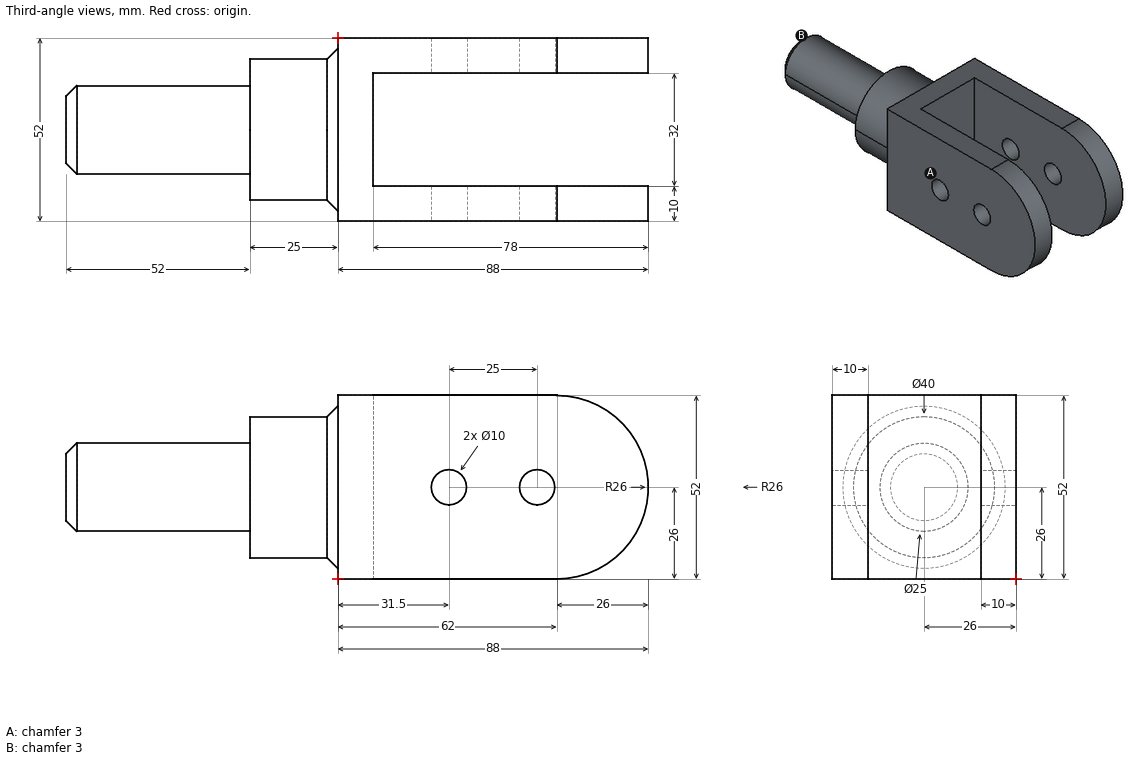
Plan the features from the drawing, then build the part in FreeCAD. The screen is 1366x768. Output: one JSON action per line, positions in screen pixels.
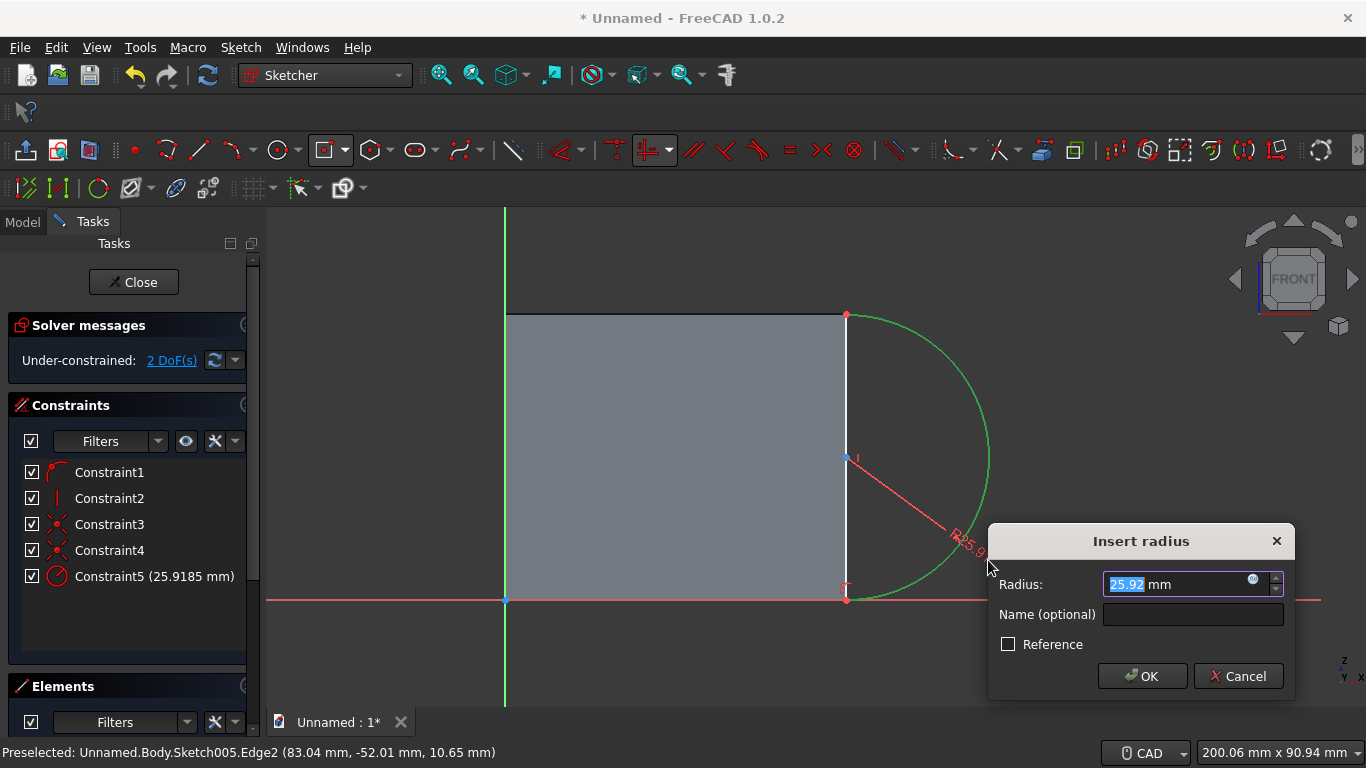
{"action": "type", "text": "26"}
{"action": "key", "text": "Return"}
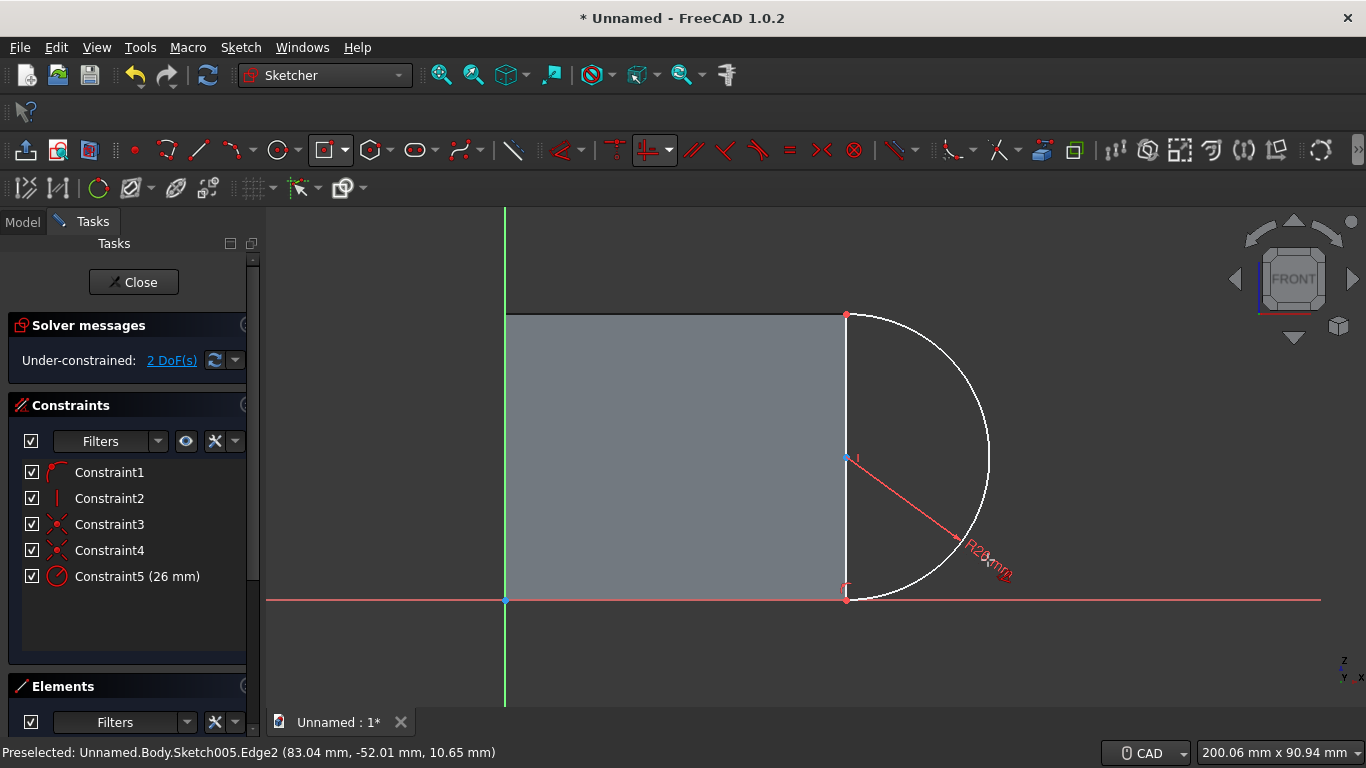
{"action": "left_click", "coordinate": [846, 314]}
{"action": "left_click", "coordinate": [676, 634]}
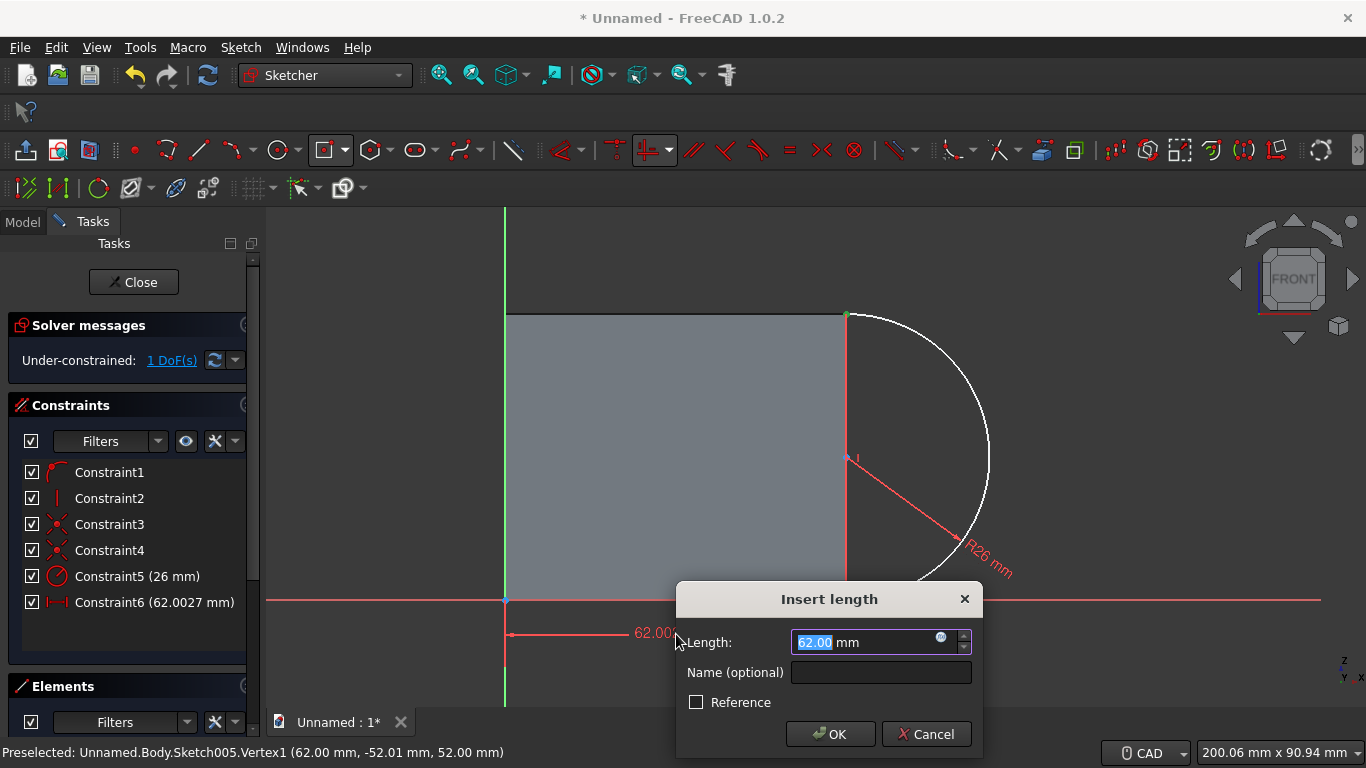
{"action": "type", "text": "62"}
{"action": "key", "text": "Return"}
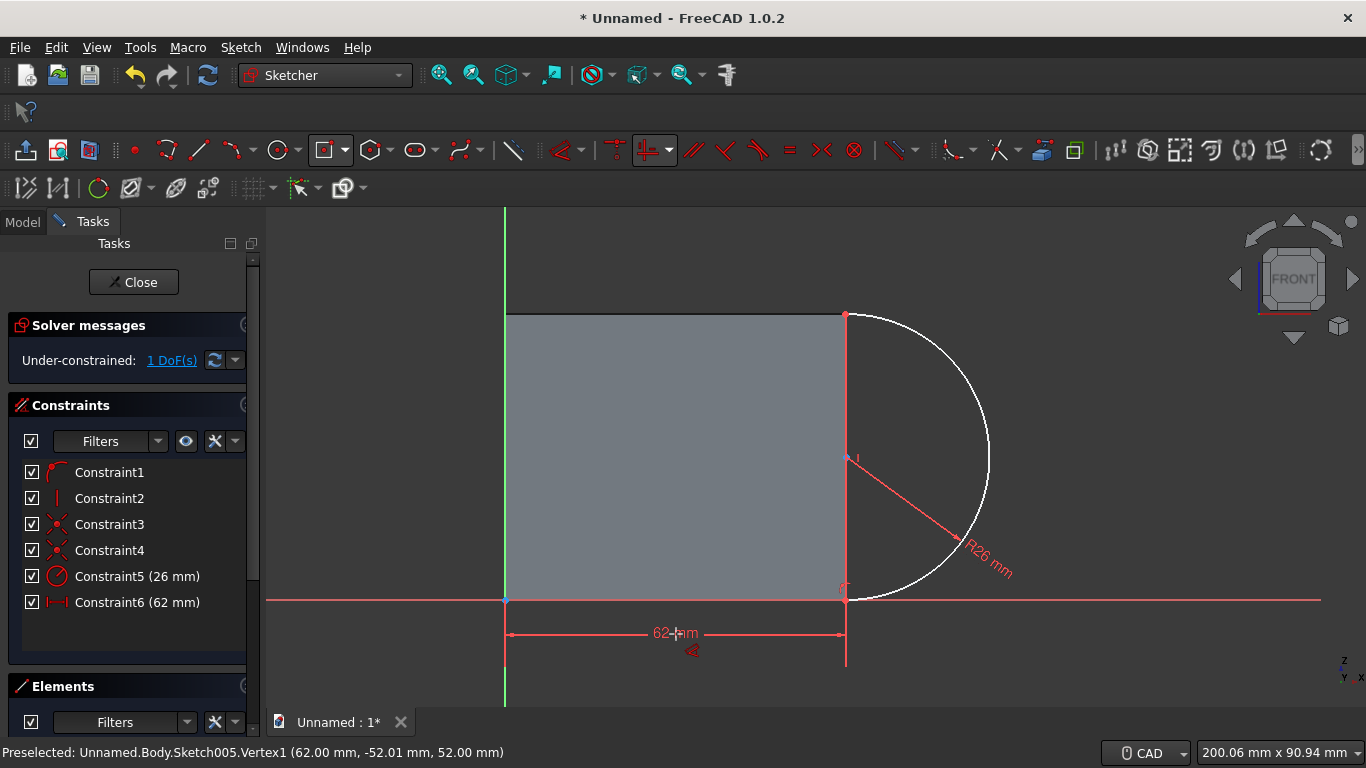
{"action": "left_click", "coordinate": [846, 457]}
{"action": "left_click", "coordinate": [597, 634]}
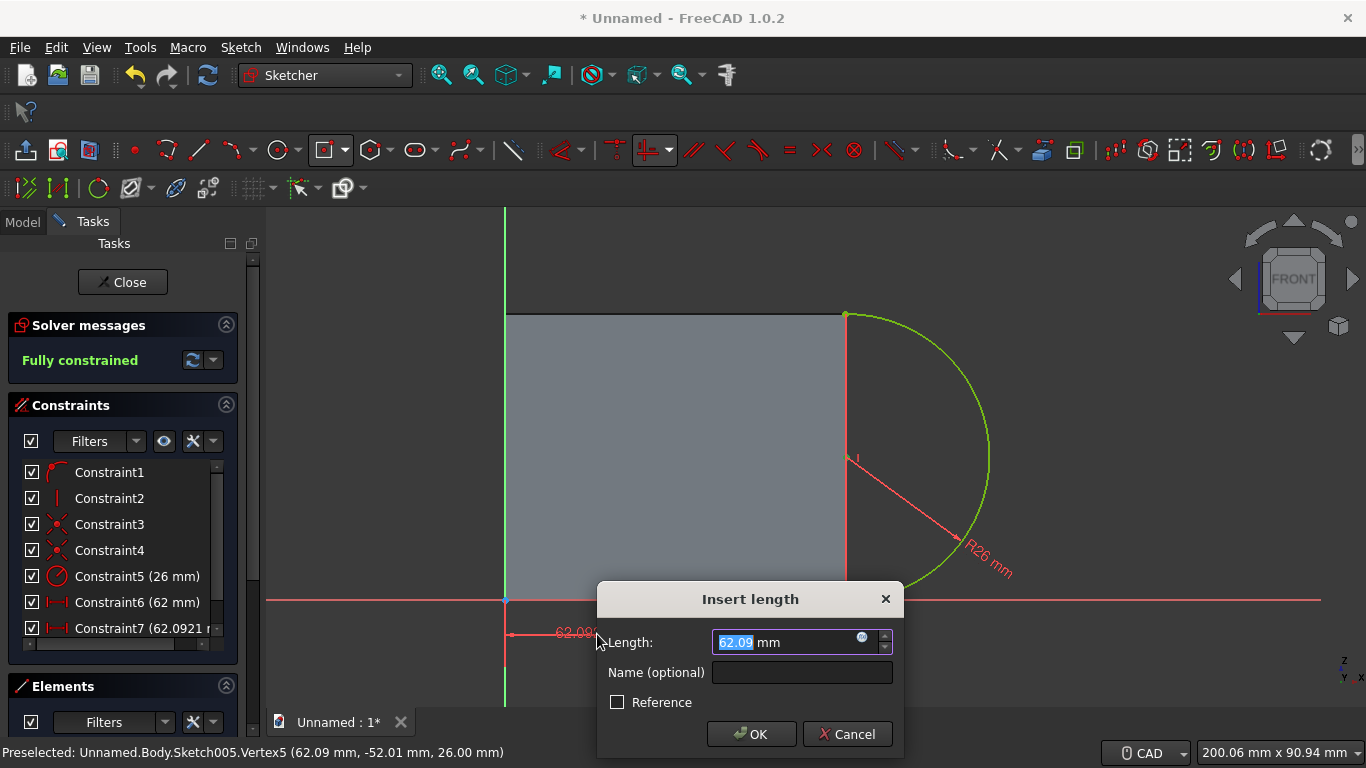
{"action": "type", "text": "62"}
{"action": "key", "text": "Return"}
{"action": "key", "text": "Escape"}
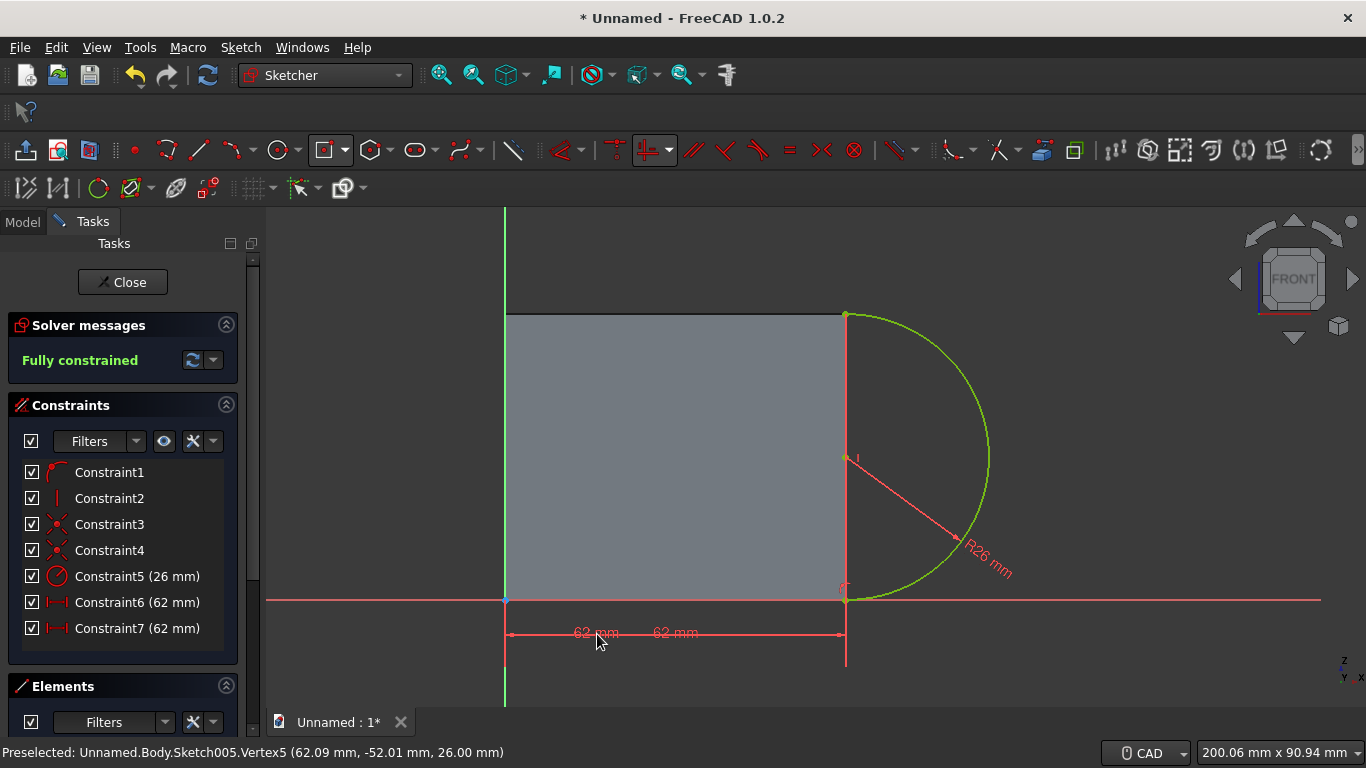
{"action": "left_click", "coordinate": [123, 282]}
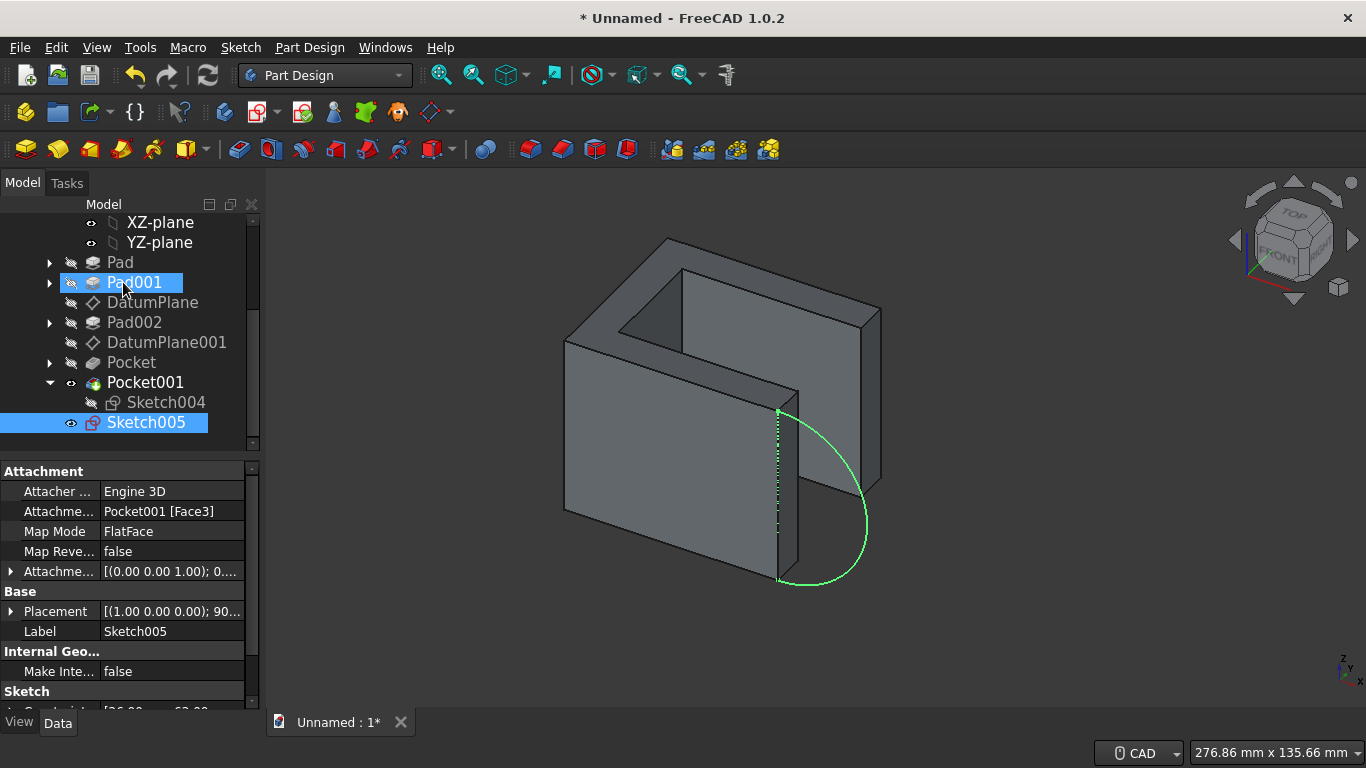
{"action": "left_click", "coordinate": [26, 150]}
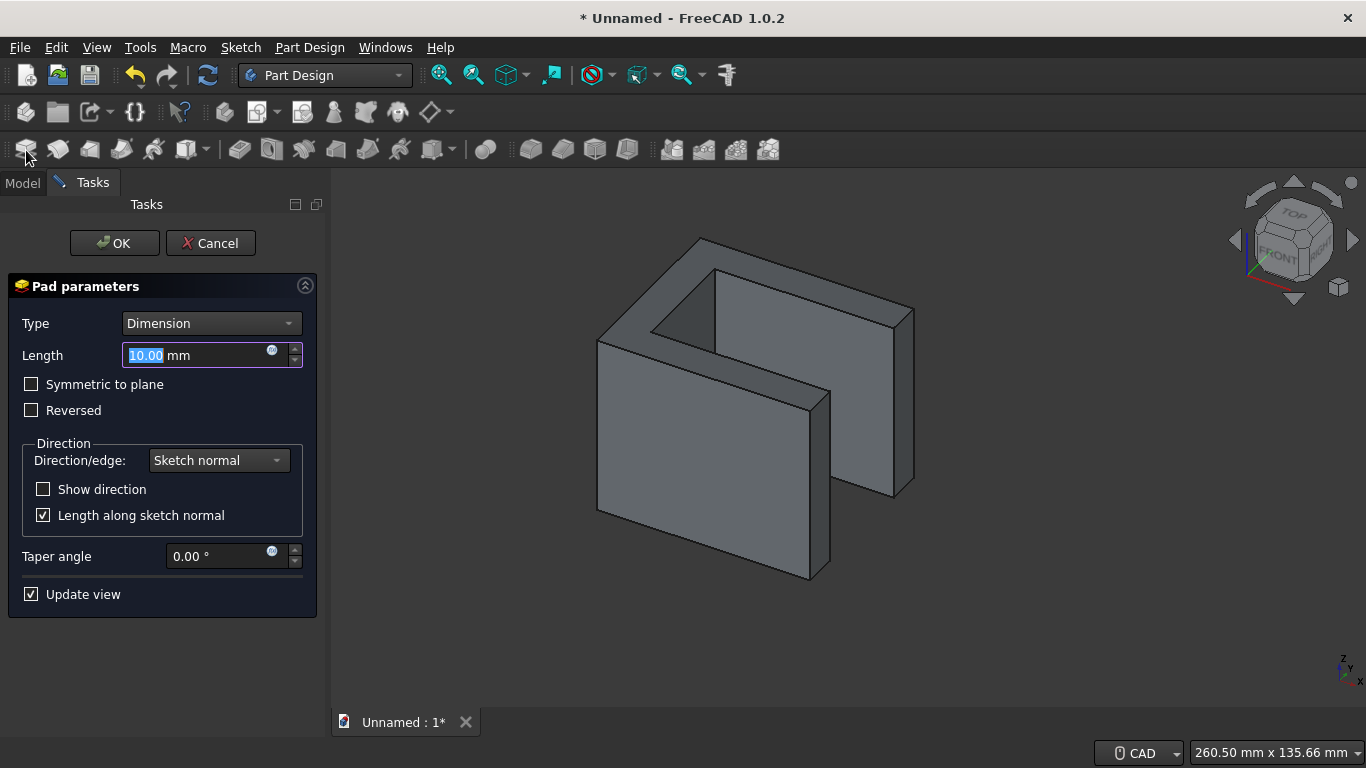
{"action": "type", "text": "10"}
{"action": "key", "text": "Tab"}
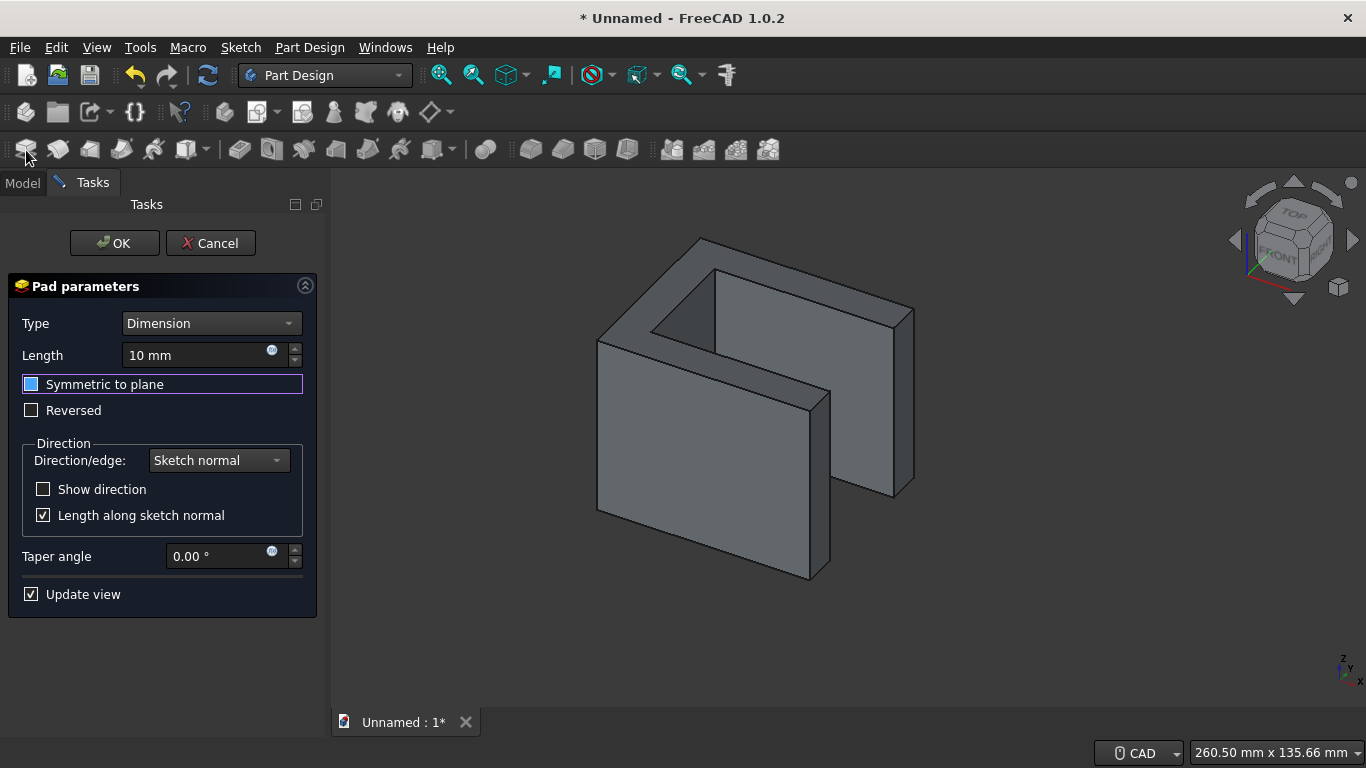
{"action": "left_click", "coordinate": [30, 410]}